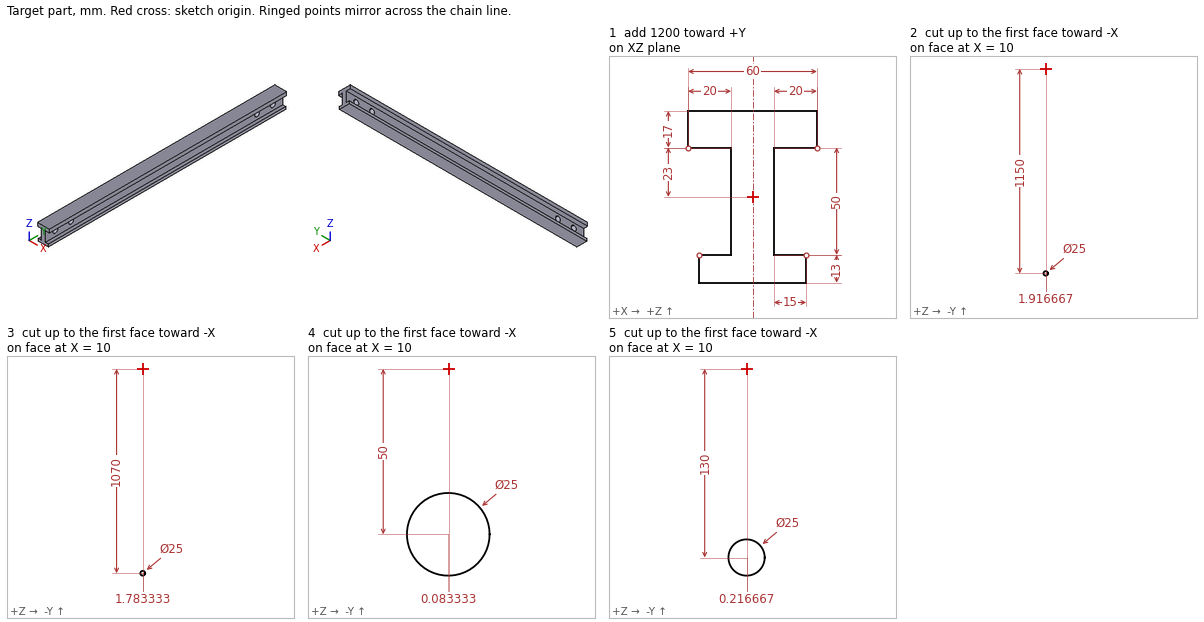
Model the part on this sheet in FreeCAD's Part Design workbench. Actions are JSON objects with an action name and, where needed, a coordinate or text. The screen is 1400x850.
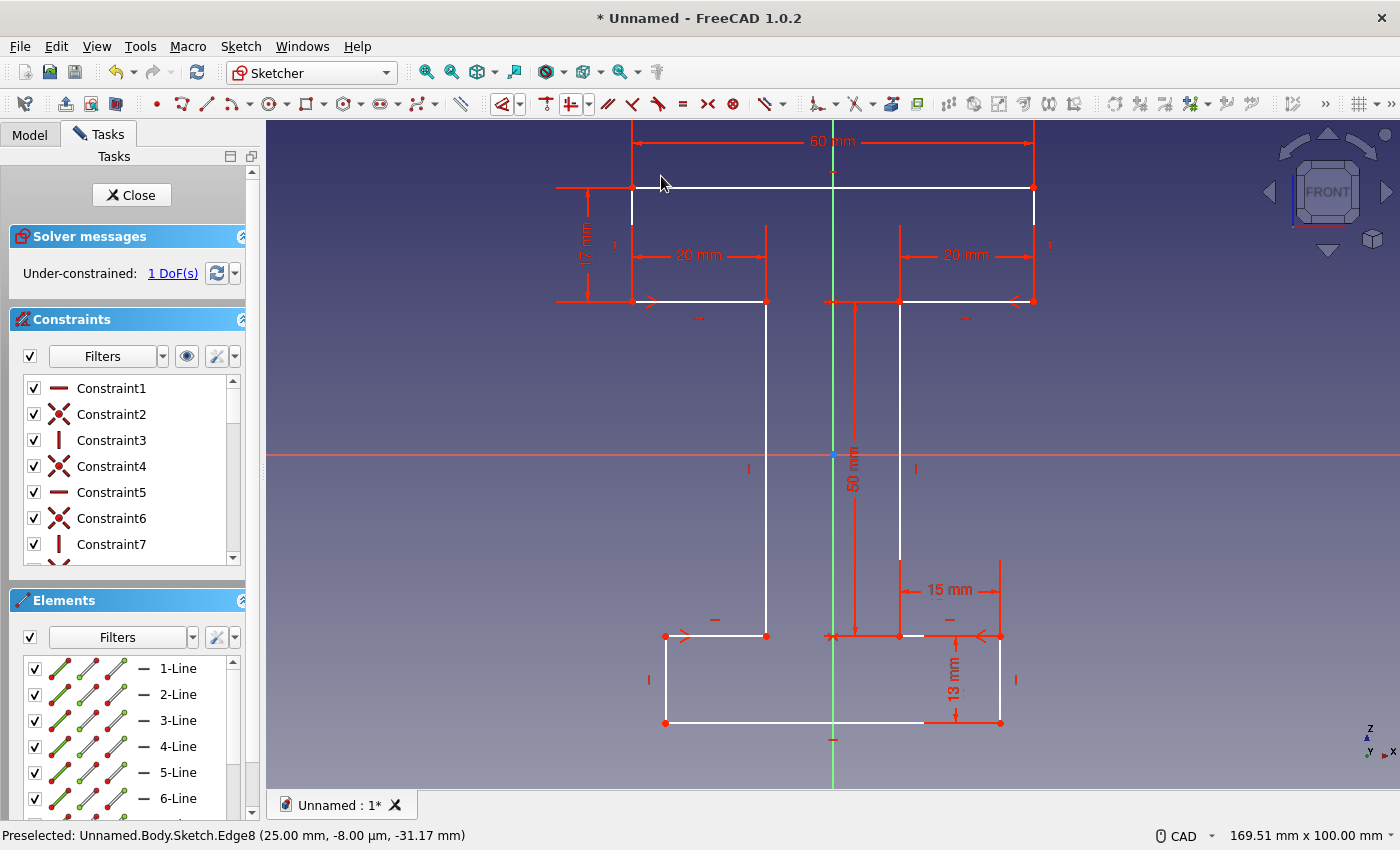
{"action": "left_click", "coordinate": [766, 302]}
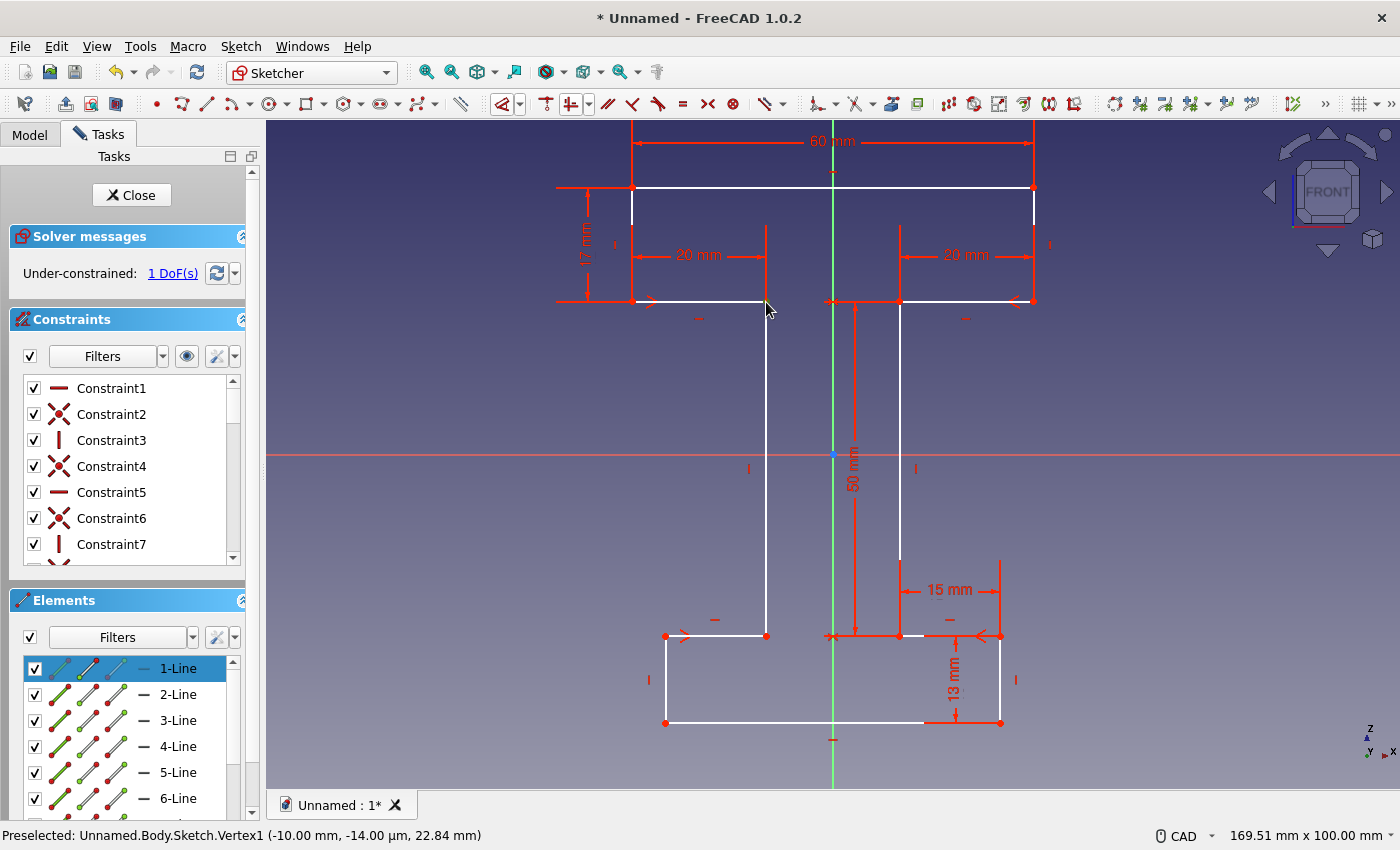
{"action": "left_click", "coordinate": [520, 104]}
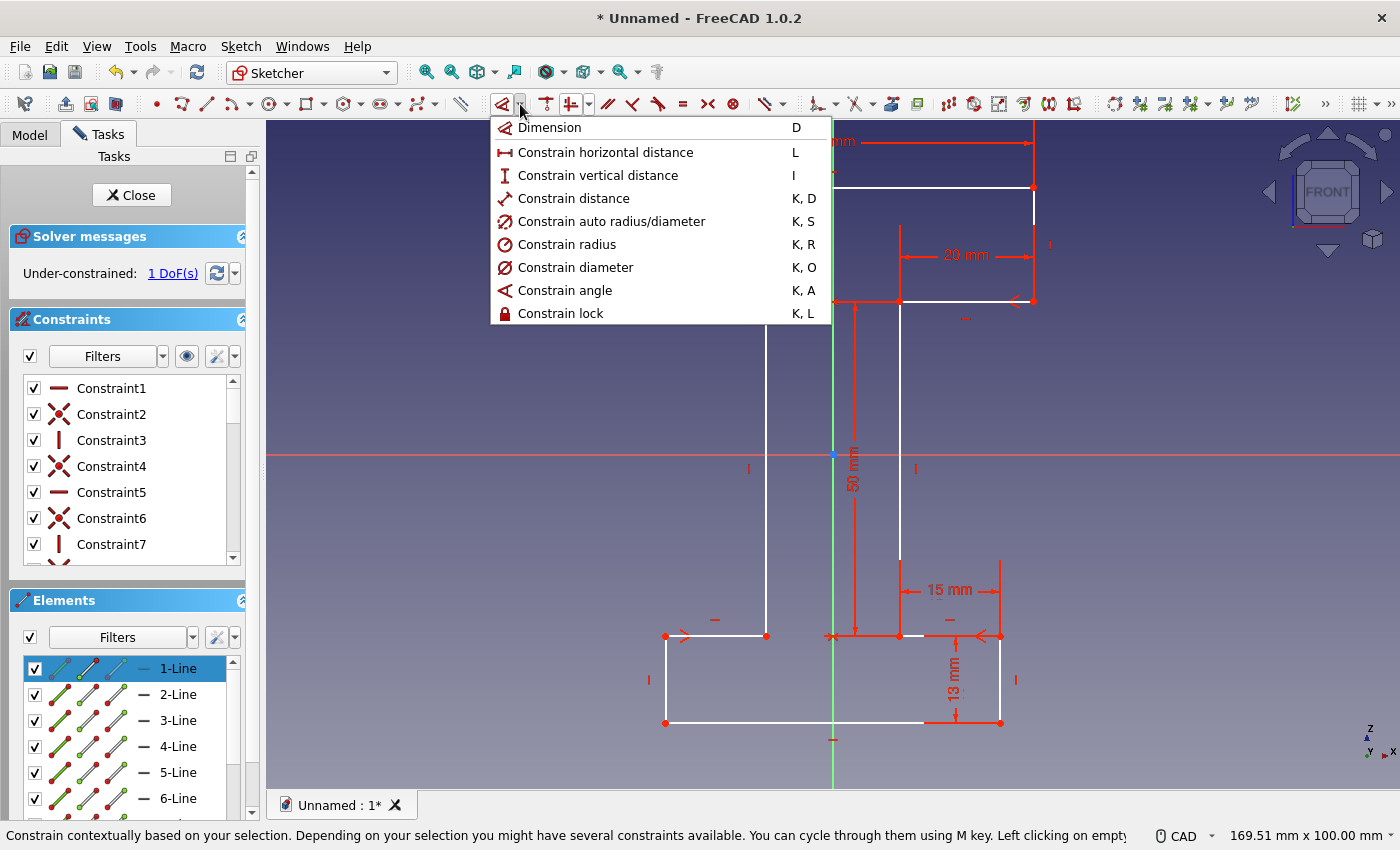
{"action": "left_click", "coordinate": [661, 176]}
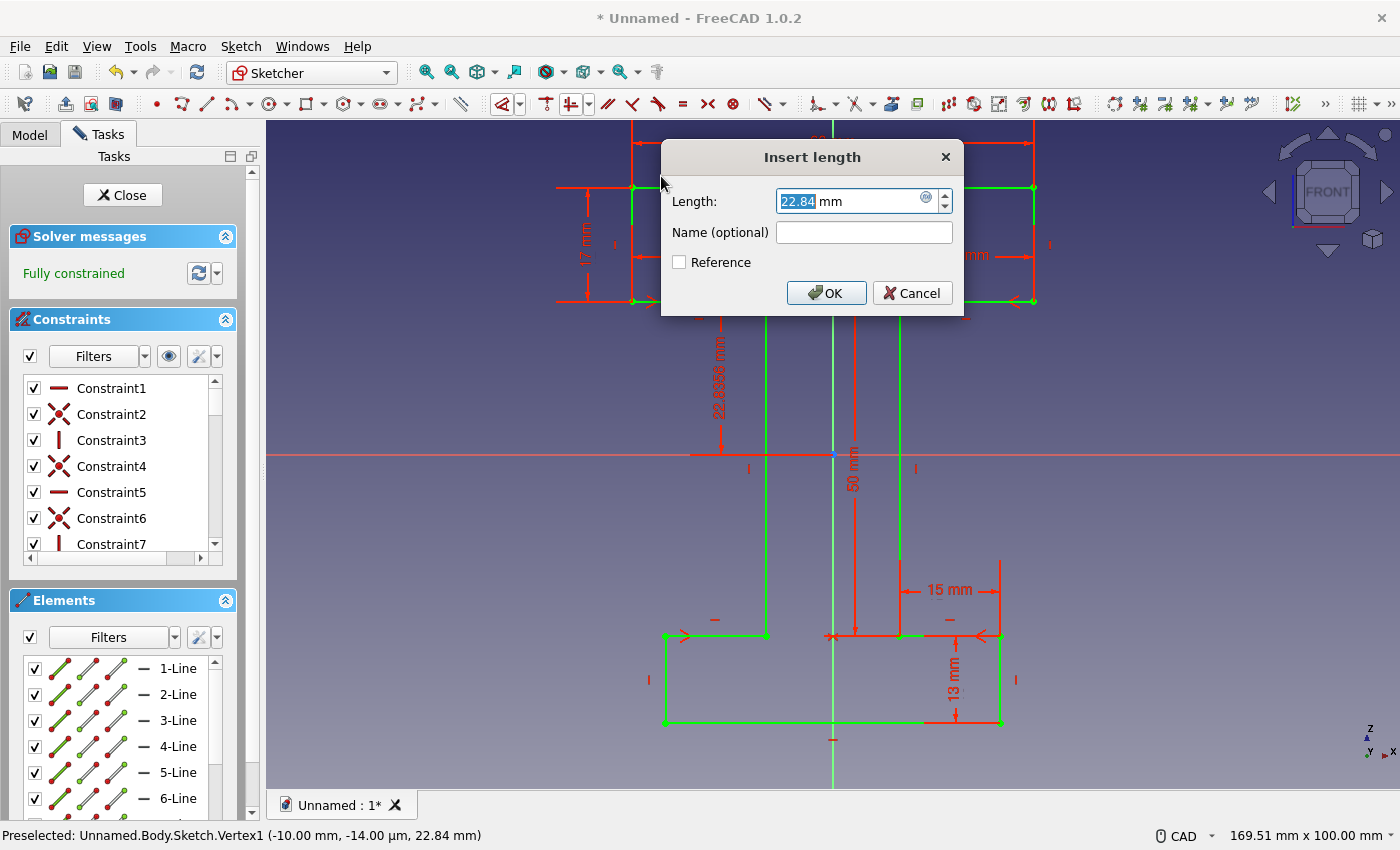
{"action": "type", "text": "23"}
{"action": "key", "text": "Return"}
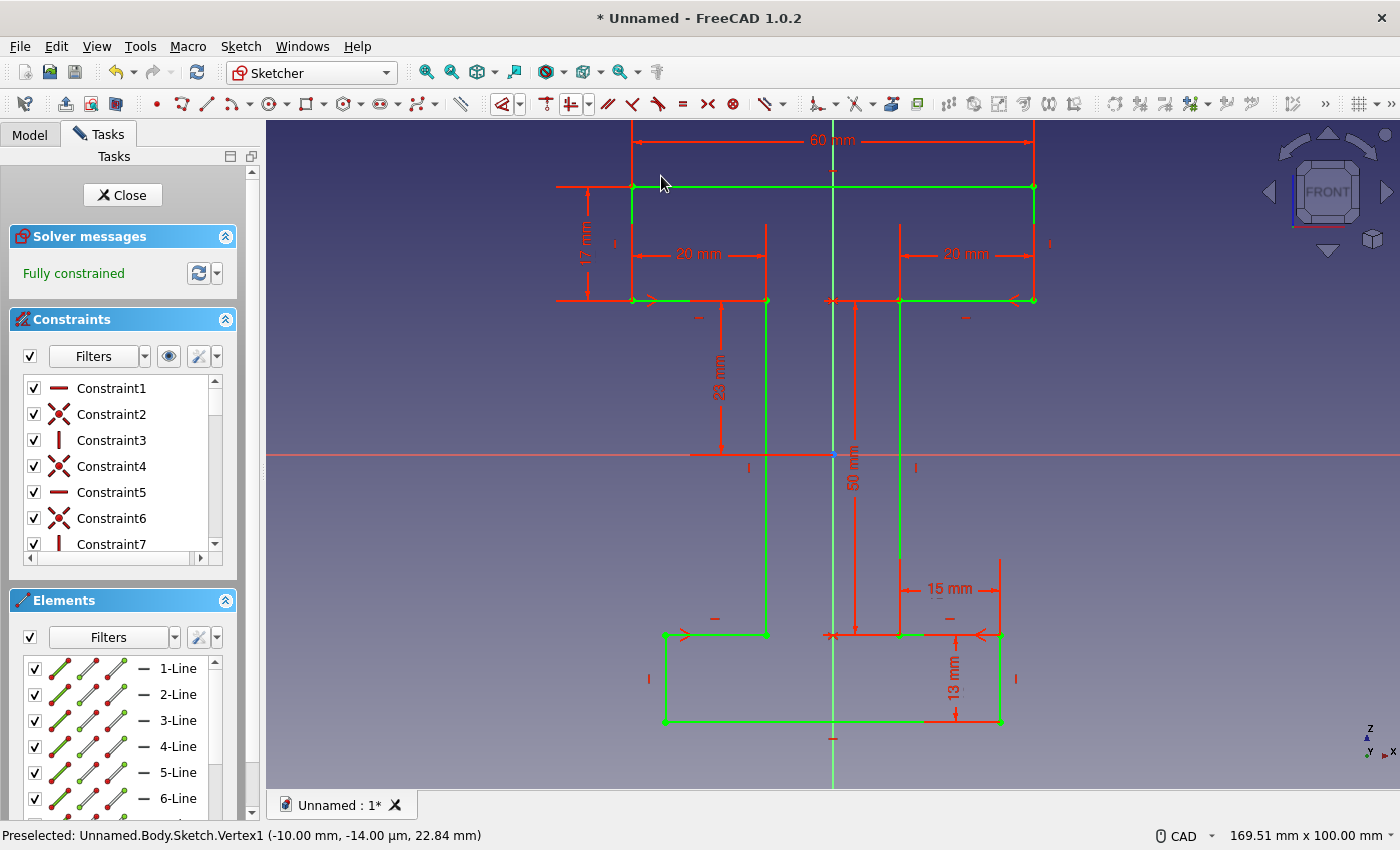
{"action": "left_click", "coordinate": [123, 195]}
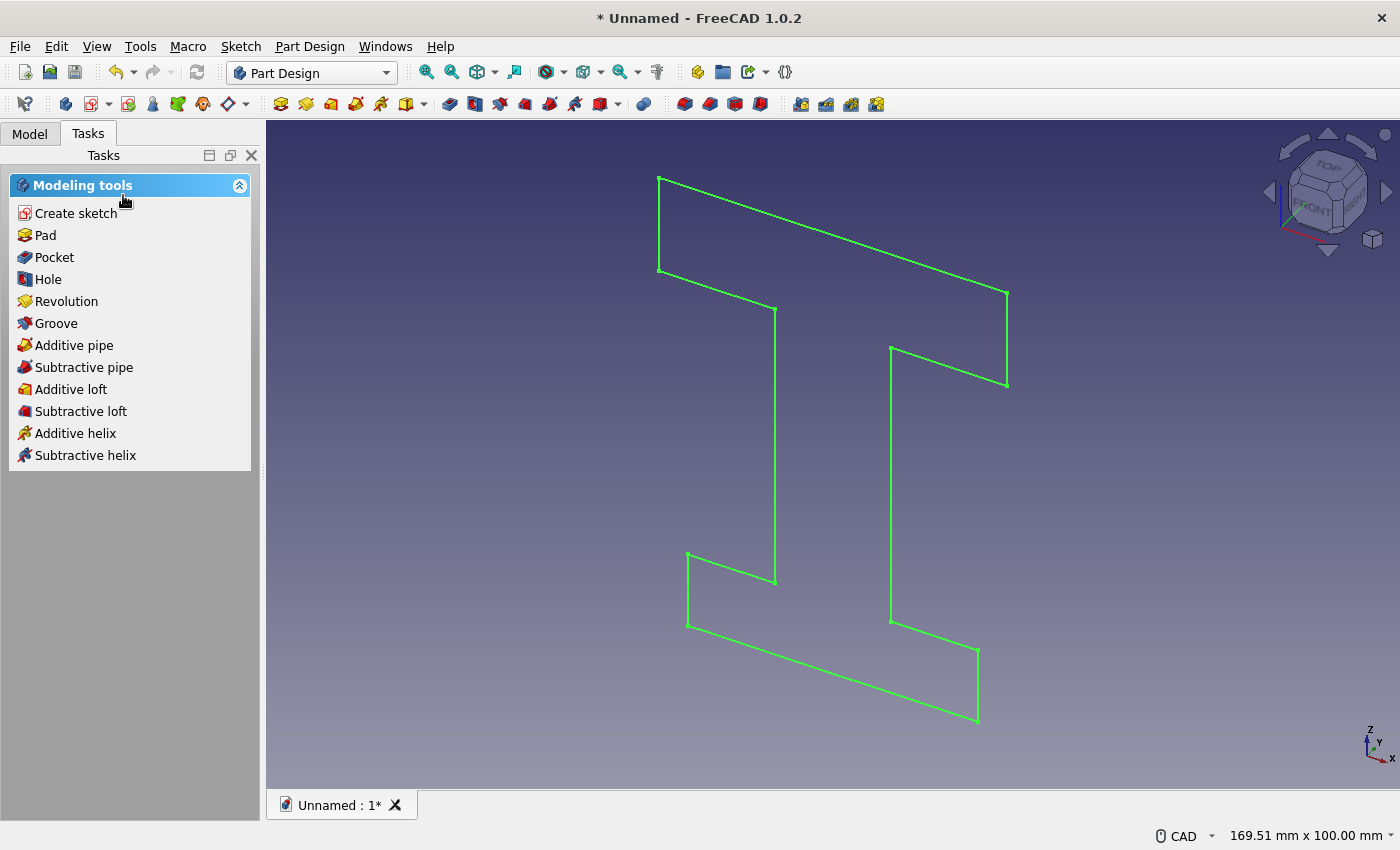
{"action": "left_click", "coordinate": [281, 104]}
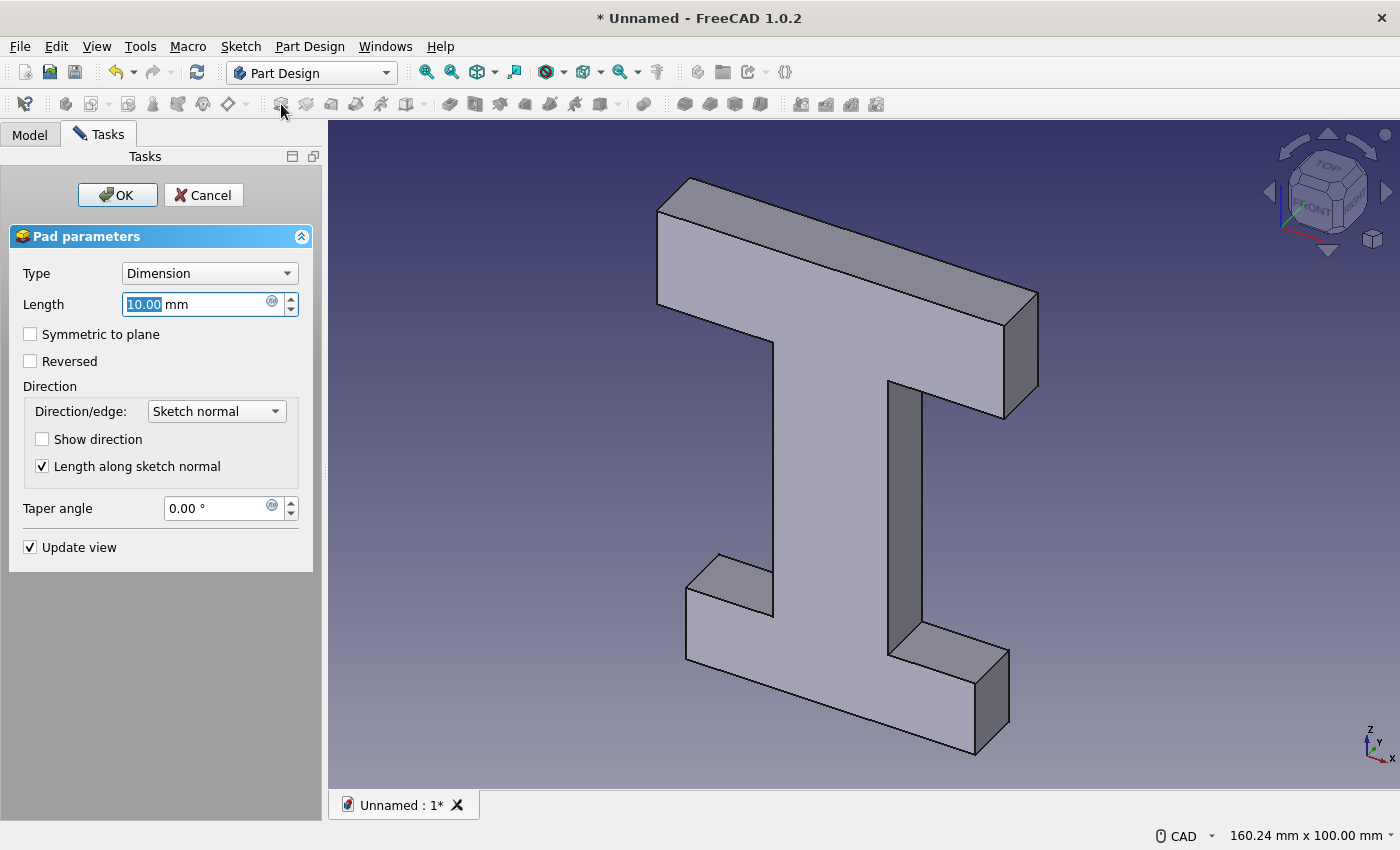
{"action": "type", "text": "1200"}
{"action": "key", "text": "Tab"}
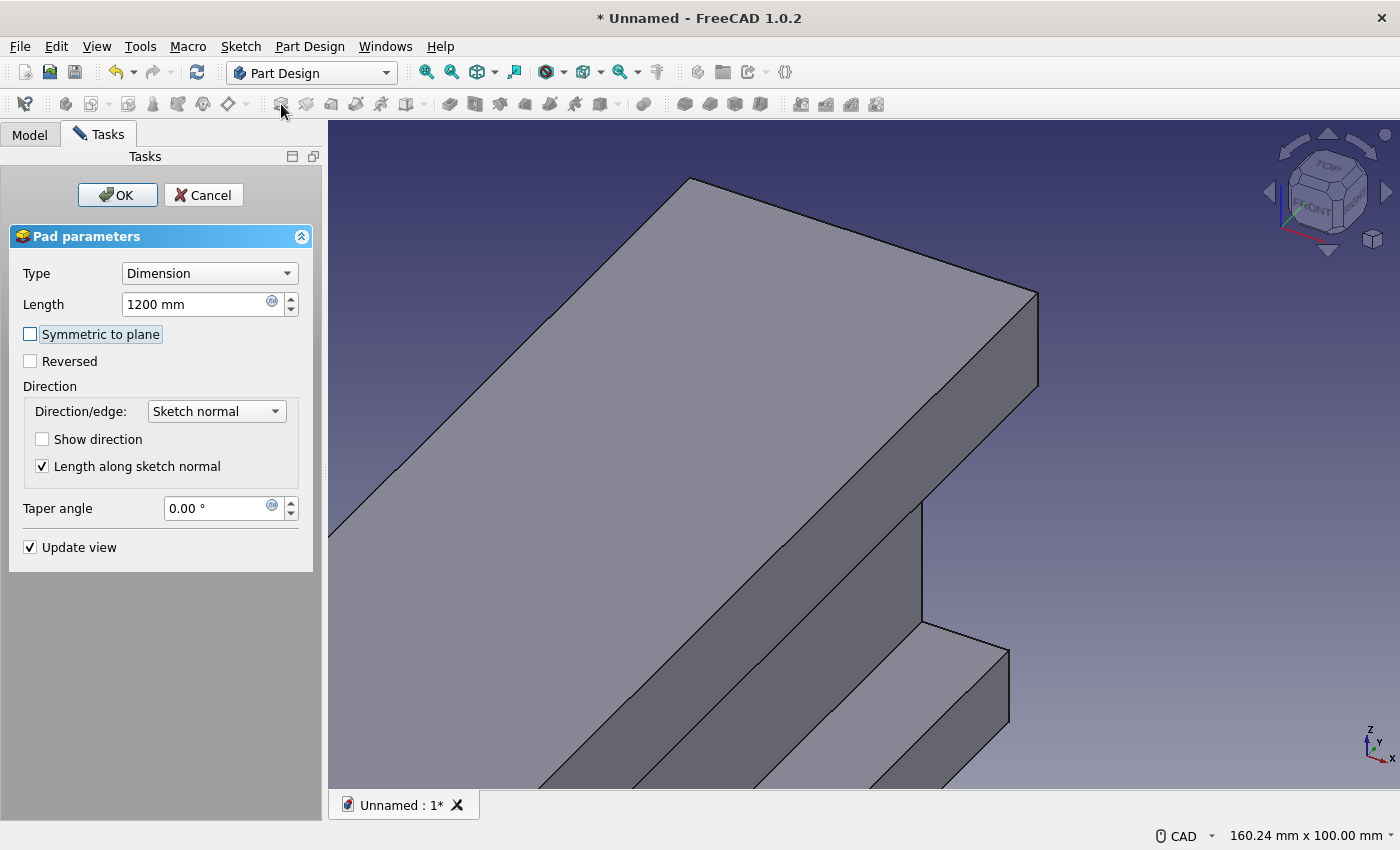
{"action": "left_click", "coordinate": [31, 361]}